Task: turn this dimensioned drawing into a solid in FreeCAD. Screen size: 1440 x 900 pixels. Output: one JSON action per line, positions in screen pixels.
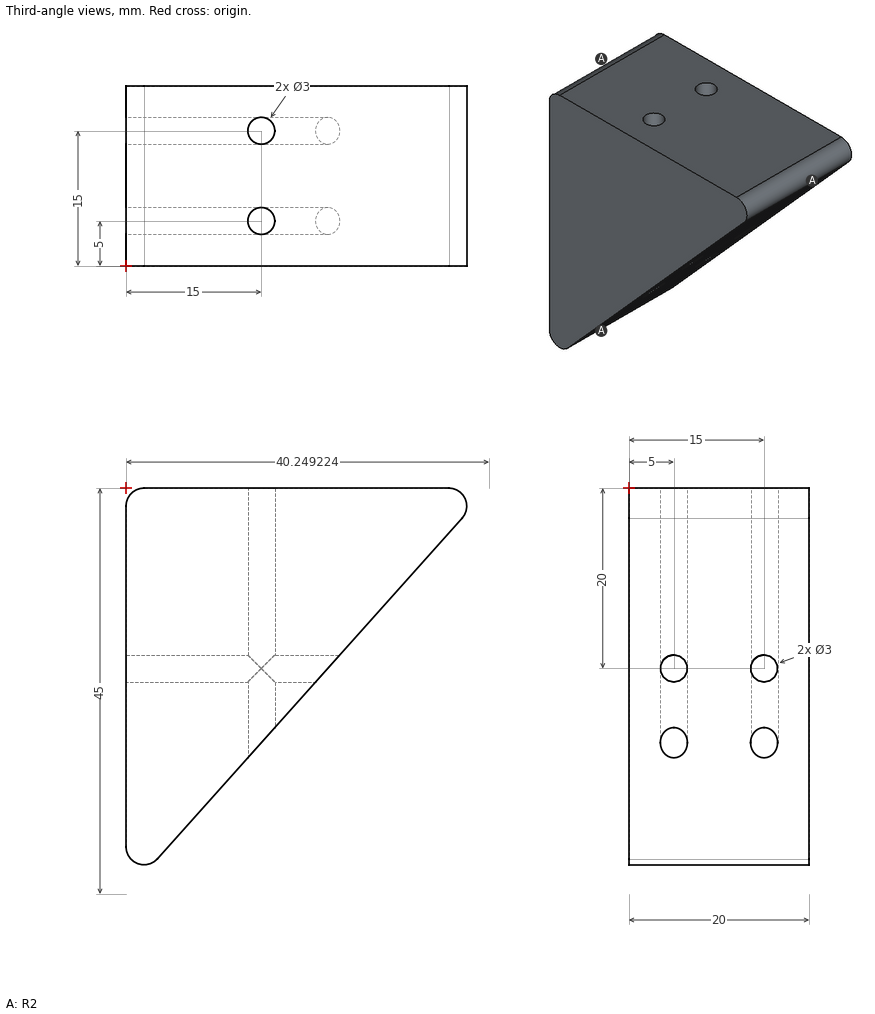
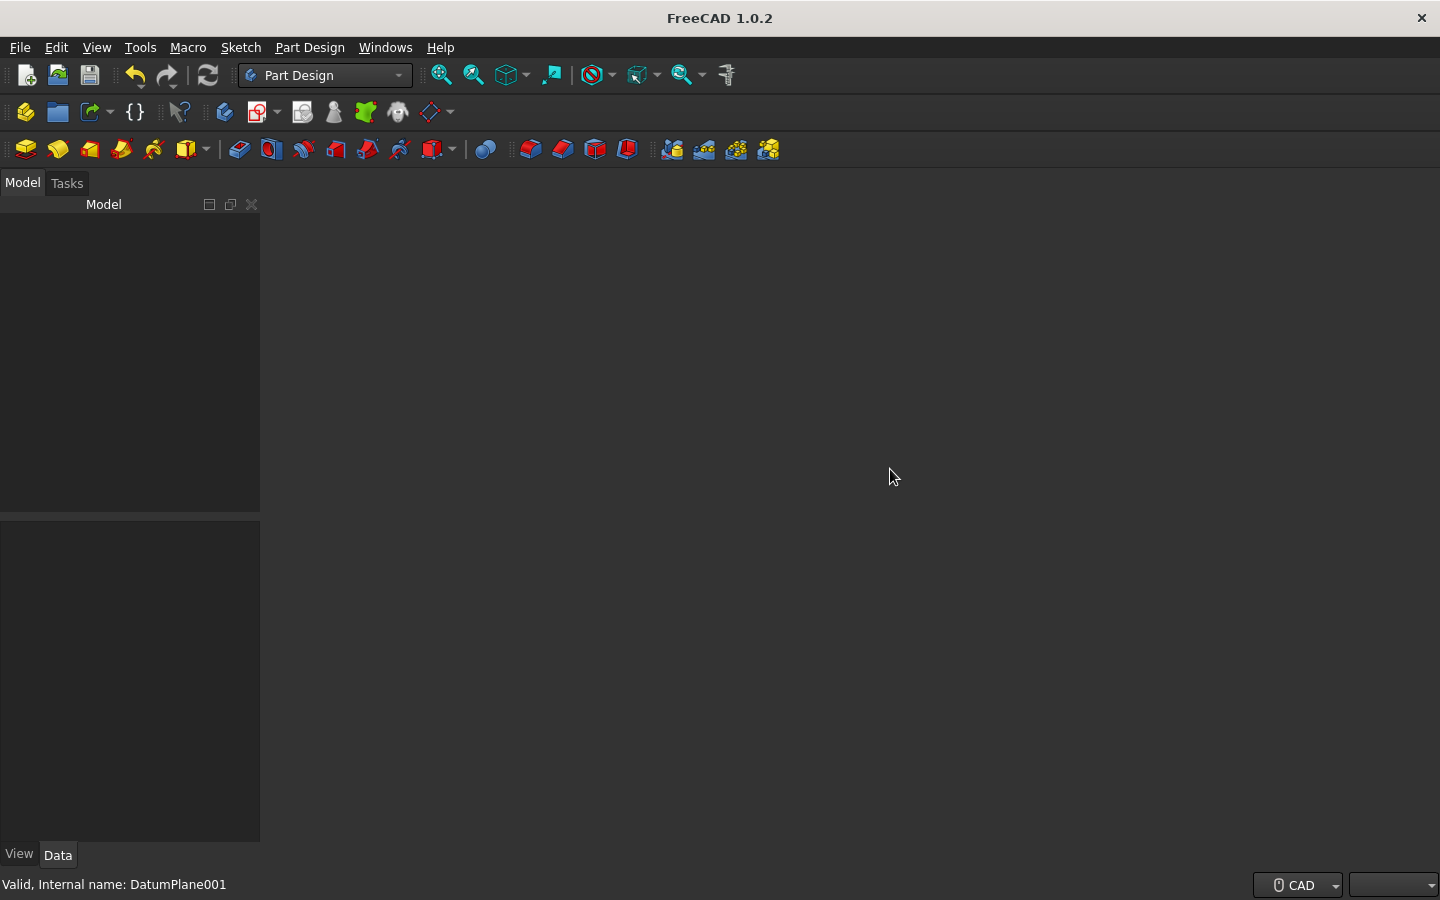
{"action": "key", "text": "ctrl+n"}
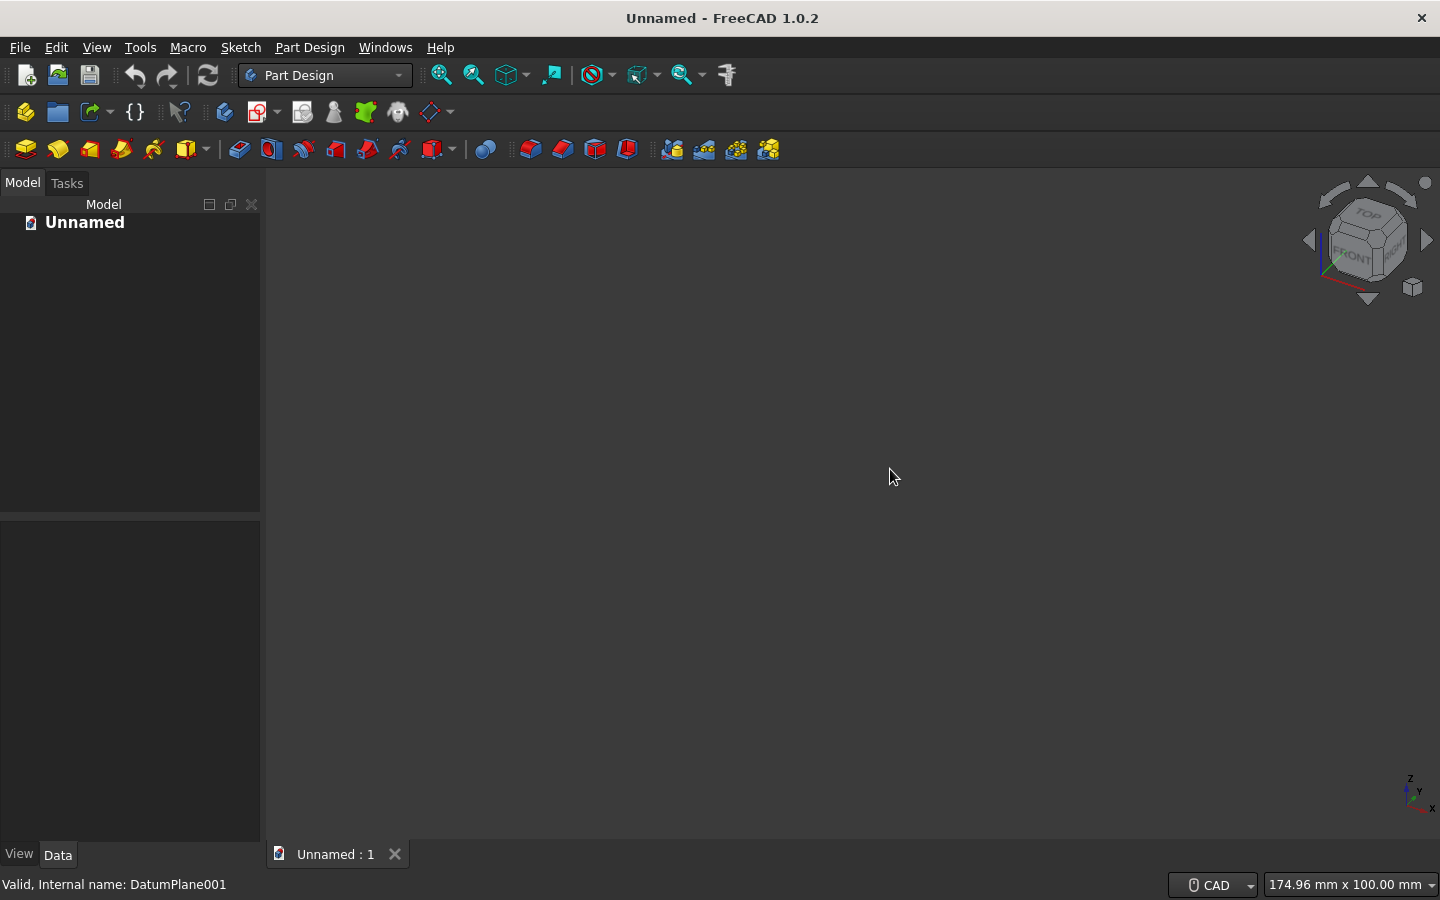
{"action": "left_click", "coordinate": [258, 112]}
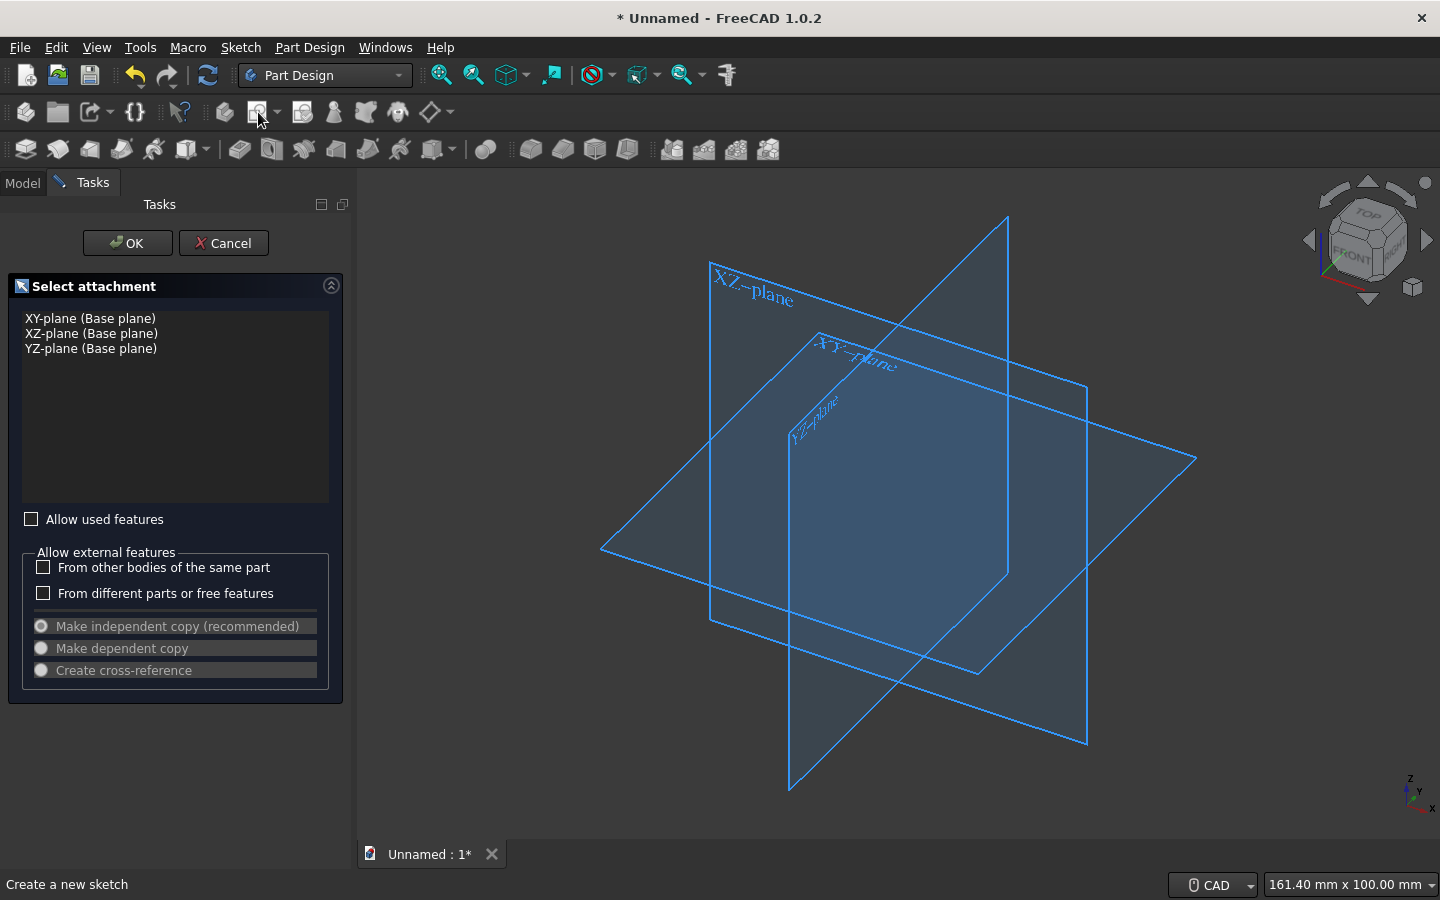
{"action": "left_click", "coordinate": [82, 334]}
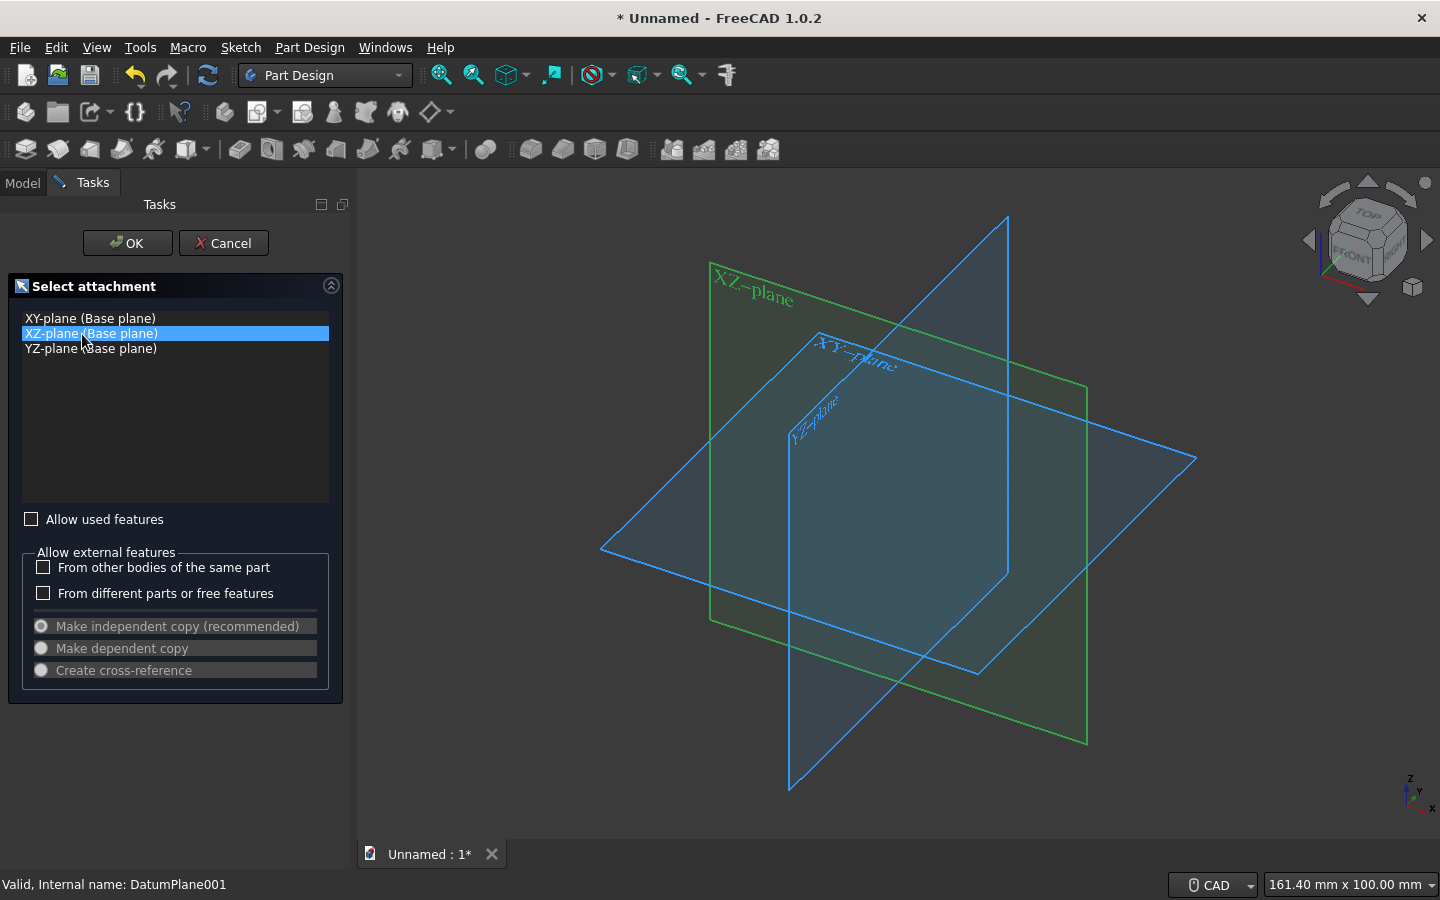
{"action": "left_click", "coordinate": [128, 243]}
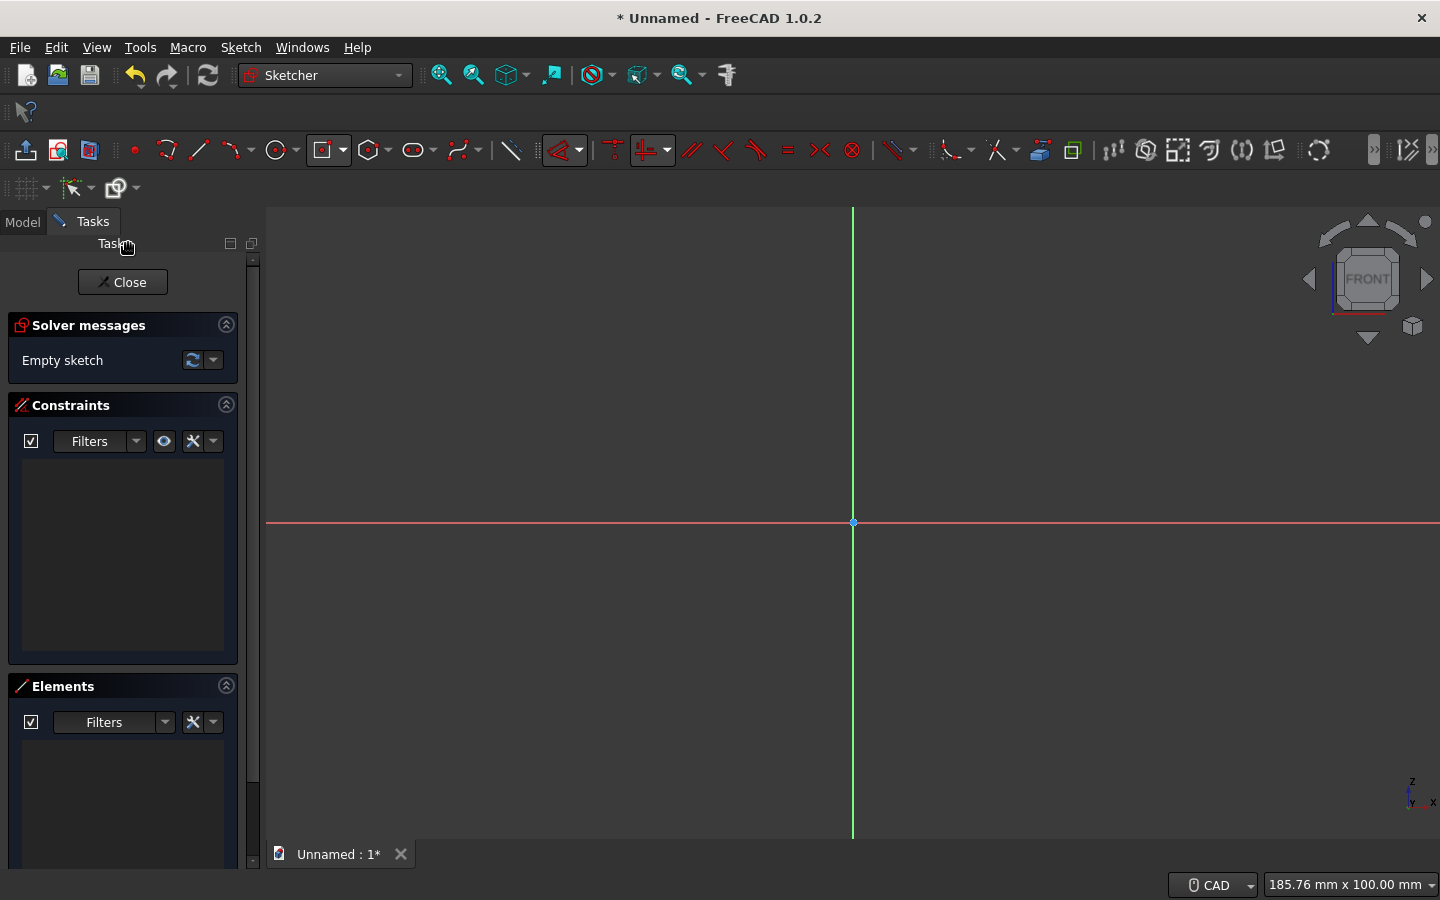
{"action": "scroll", "coordinate": [294, 235], "scroll_direction": "down", "scroll_amount": 1}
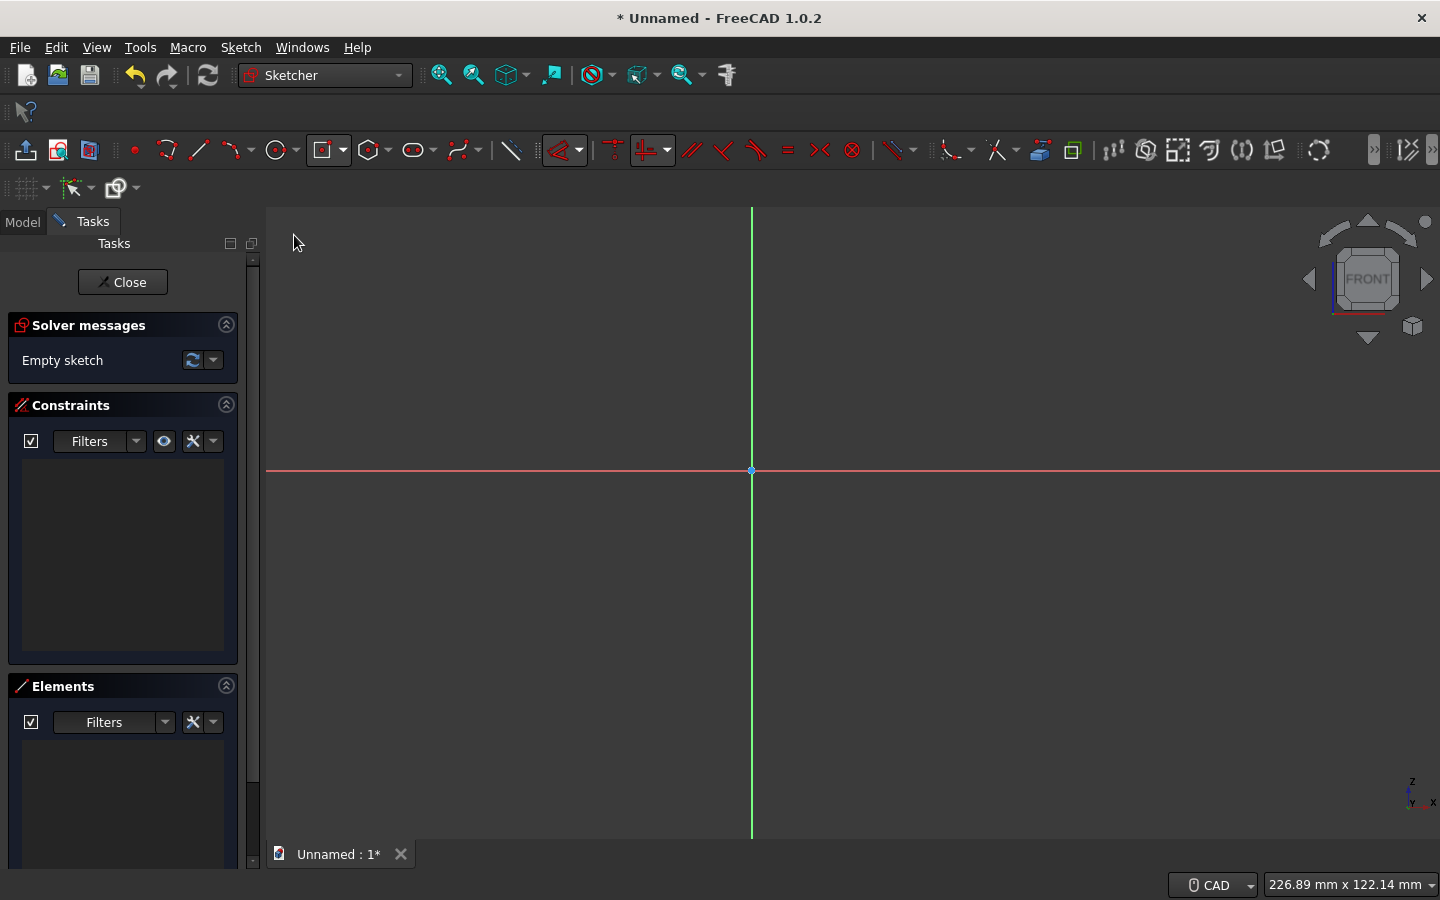
{"action": "scroll", "coordinate": [943, 665], "scroll_direction": "up", "scroll_amount": 3}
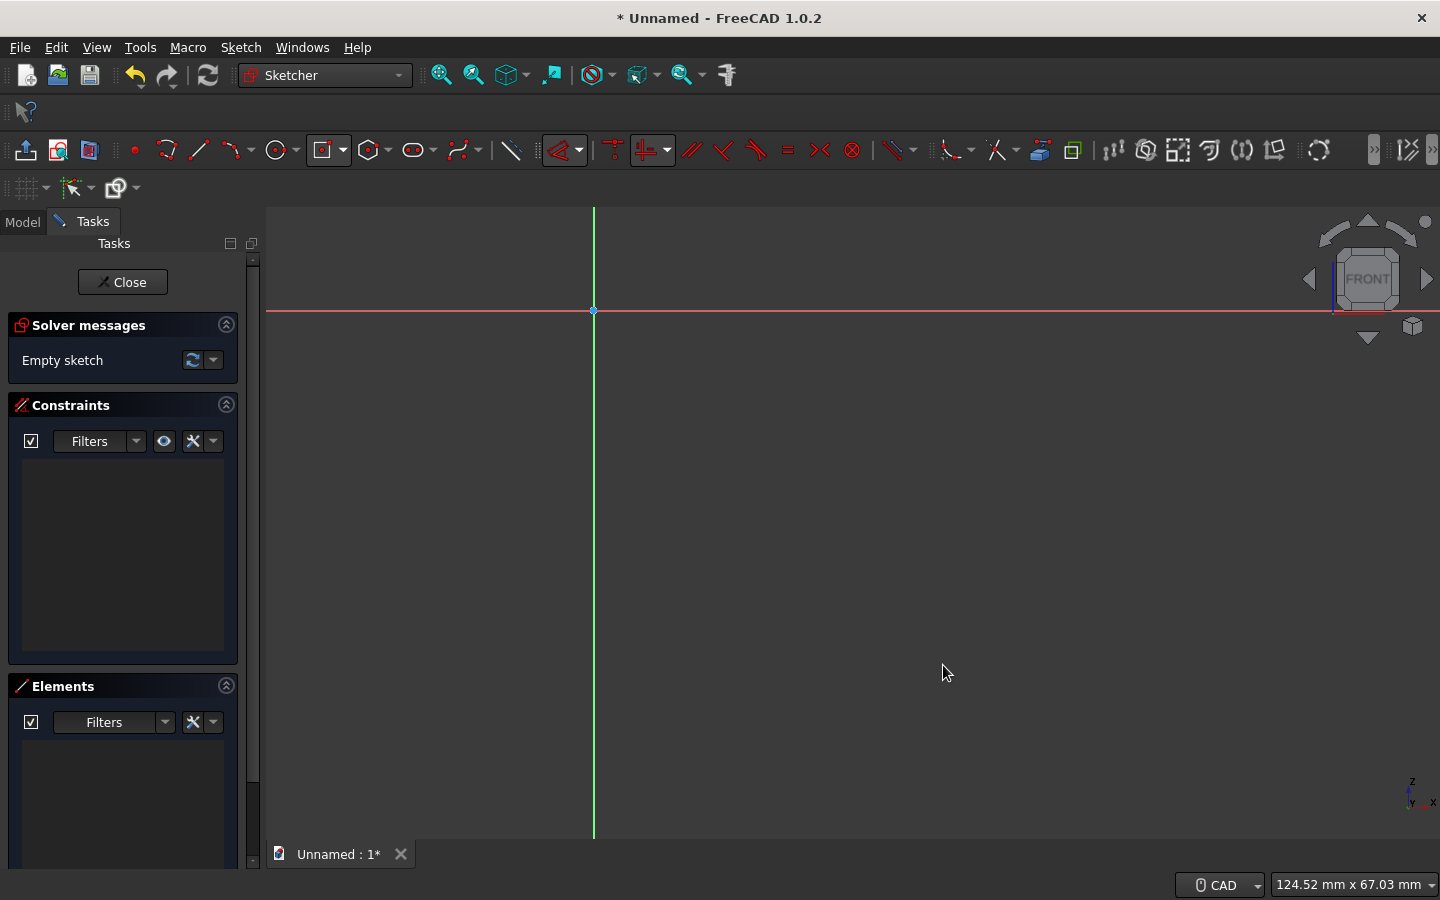
{"action": "left_click", "coordinate": [168, 150]}